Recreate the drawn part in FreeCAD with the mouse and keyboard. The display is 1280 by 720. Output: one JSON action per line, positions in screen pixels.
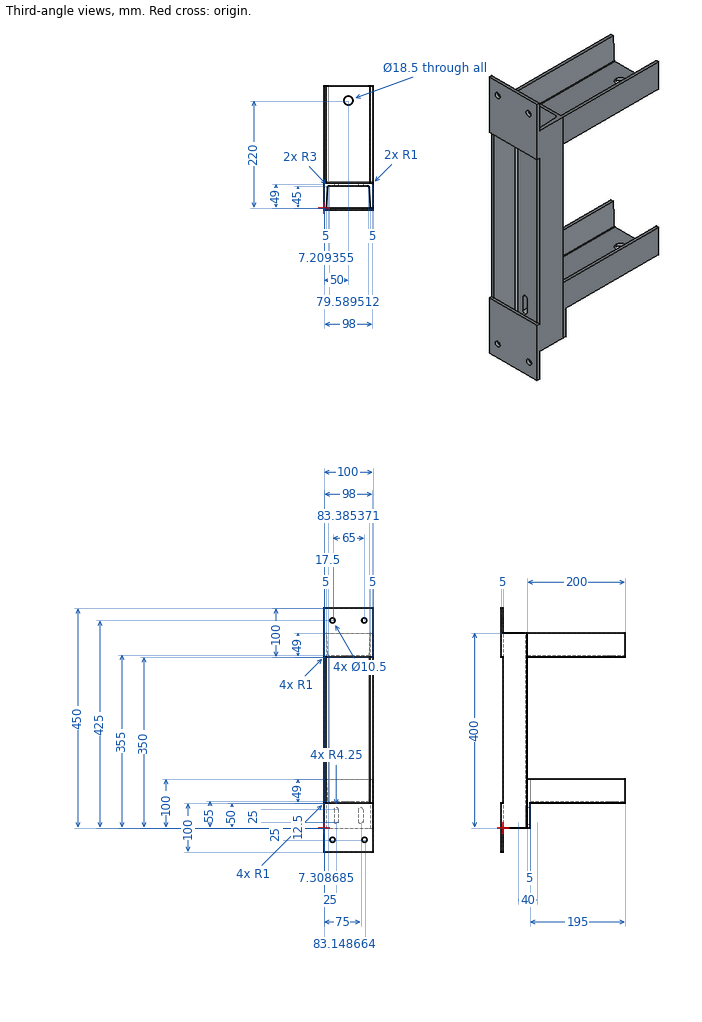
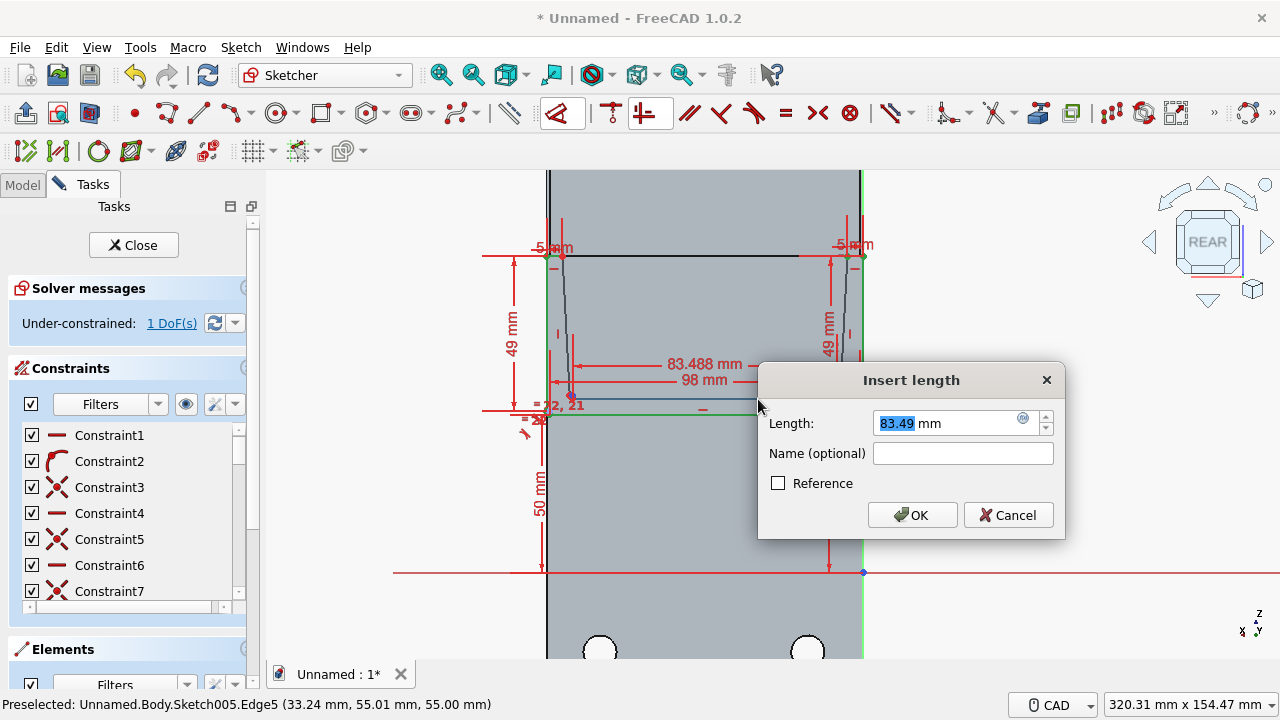
{"action": "type", "text": "83.385371"}
{"action": "key", "text": "Return"}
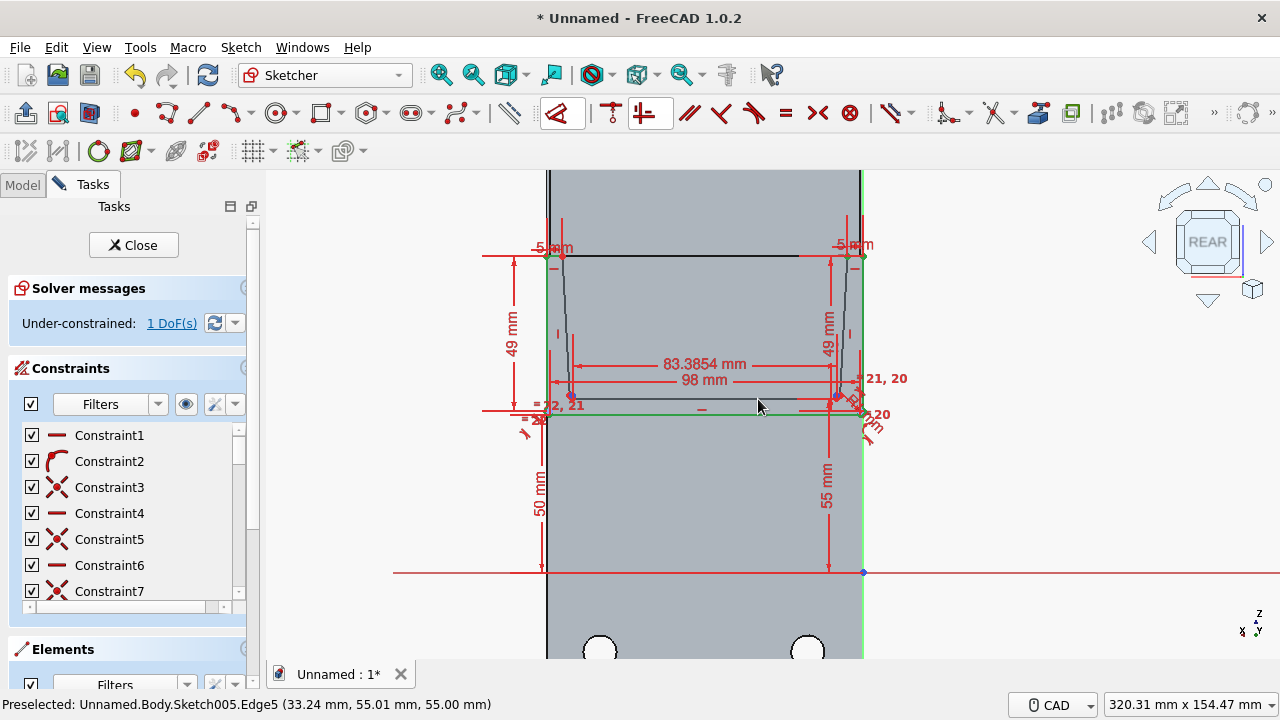
{"action": "scroll", "coordinate": [840, 396], "scroll_direction": "up", "scroll_amount": 7}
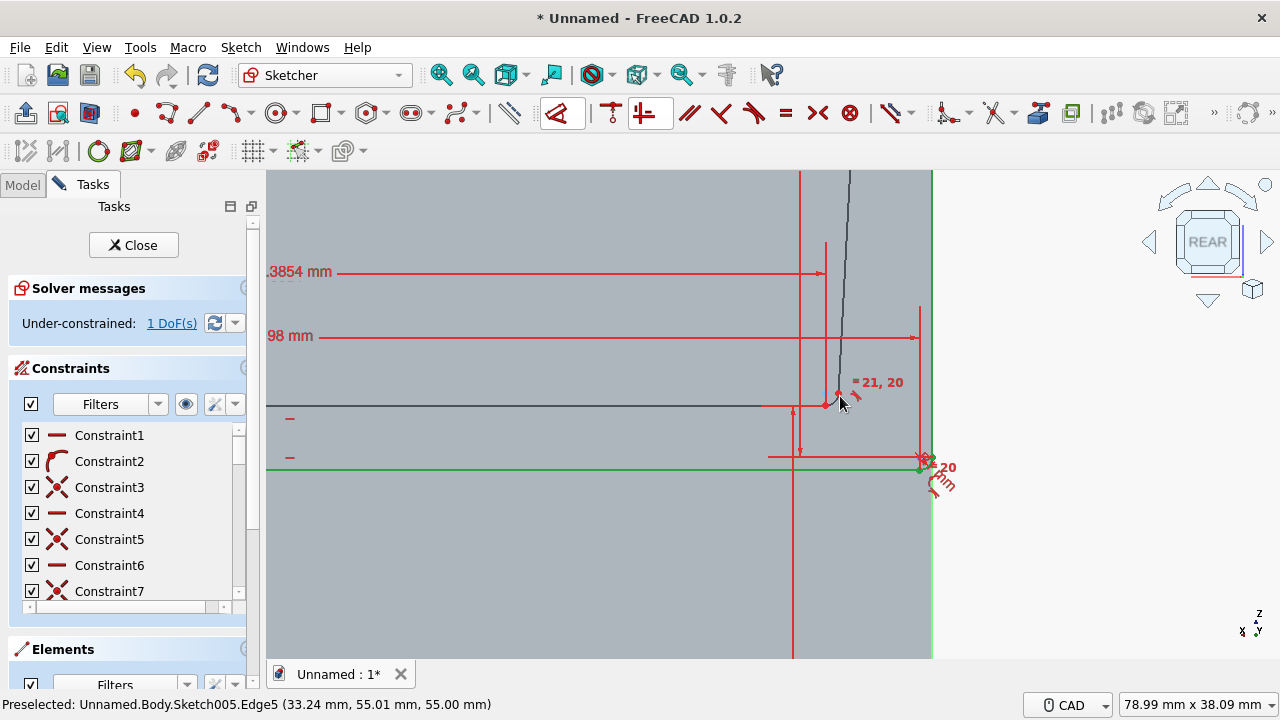
{"action": "left_click", "coordinate": [838, 394]}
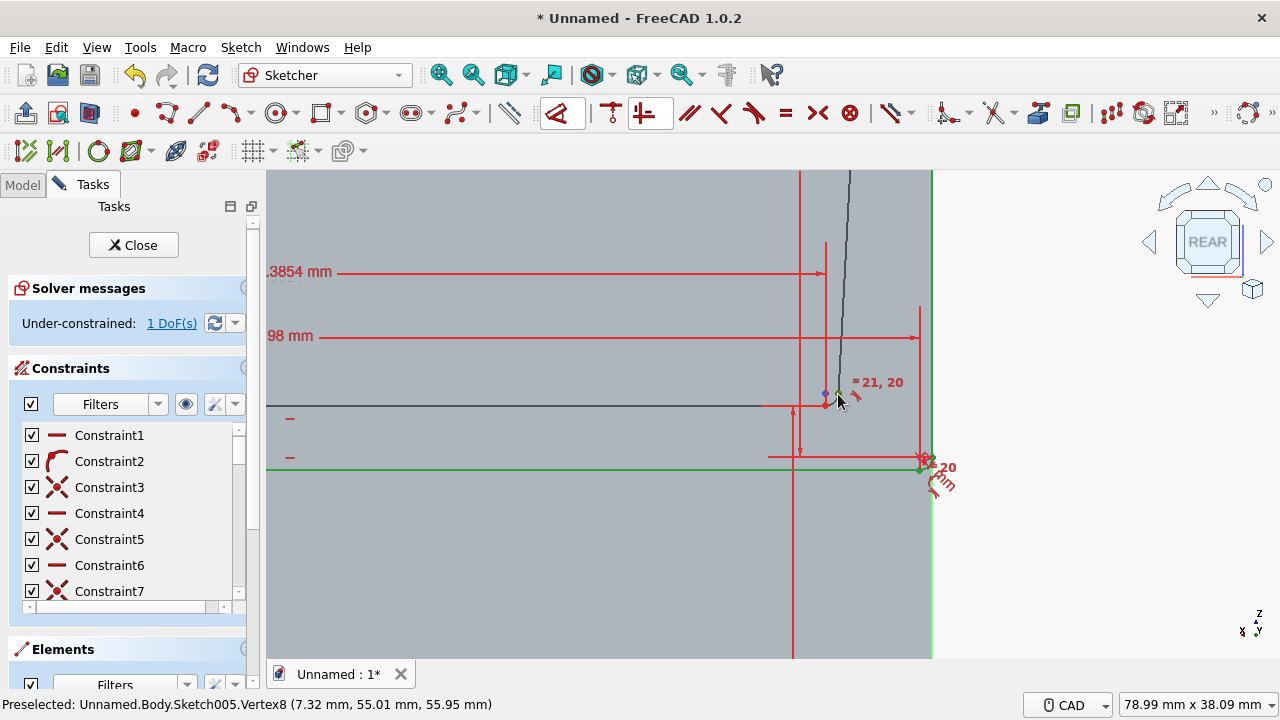
{"action": "key", "text": "l"}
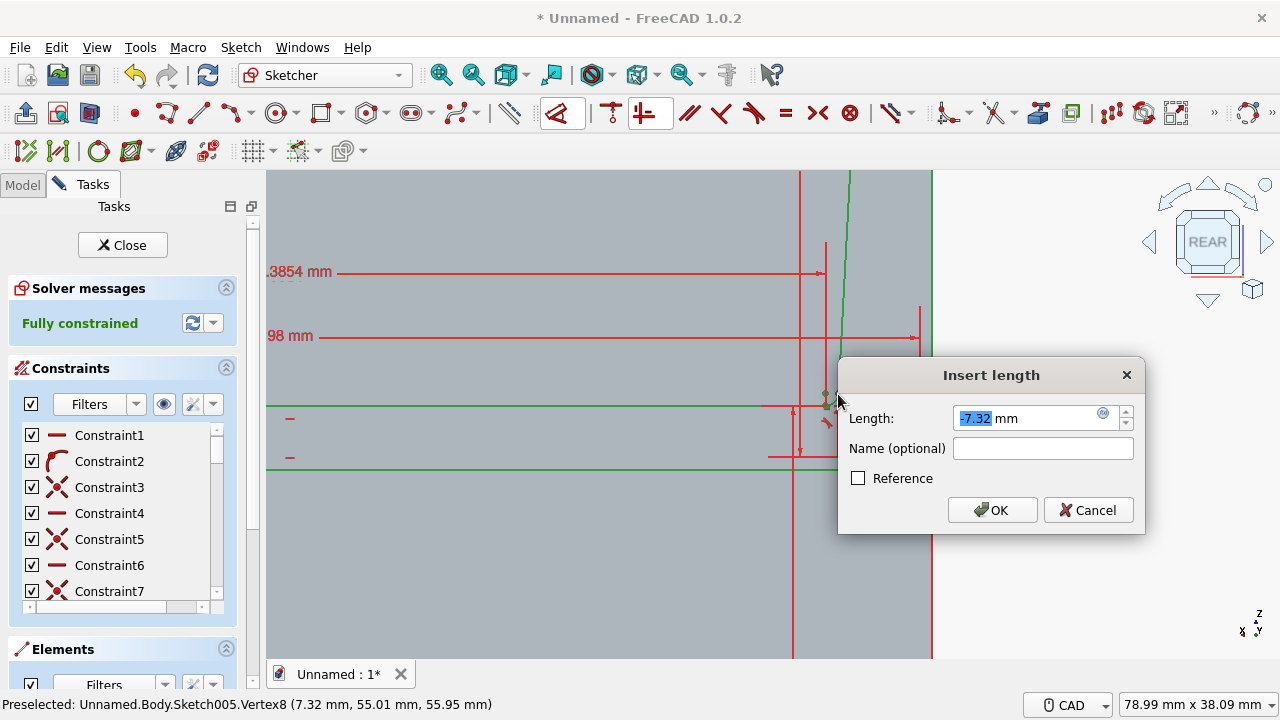
{"action": "type", "text": "-7.308685"}
{"action": "key", "text": "Return"}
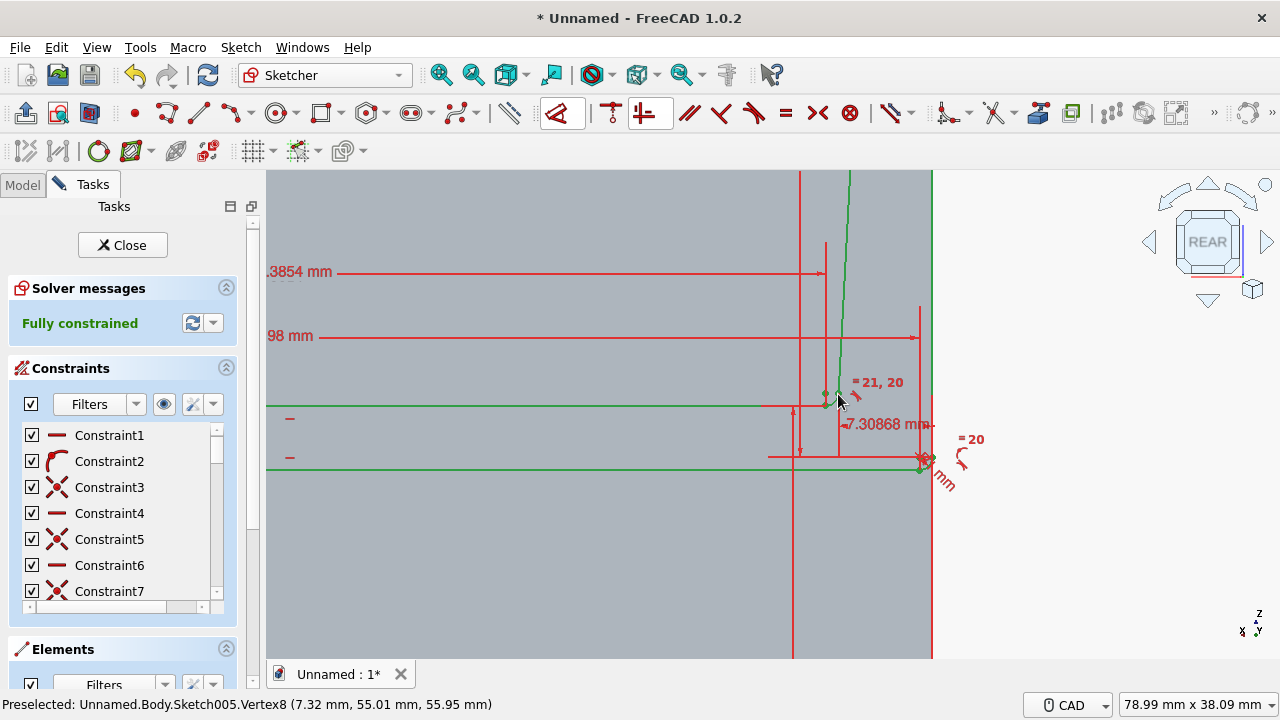
{"action": "left_click", "coordinate": [123, 245]}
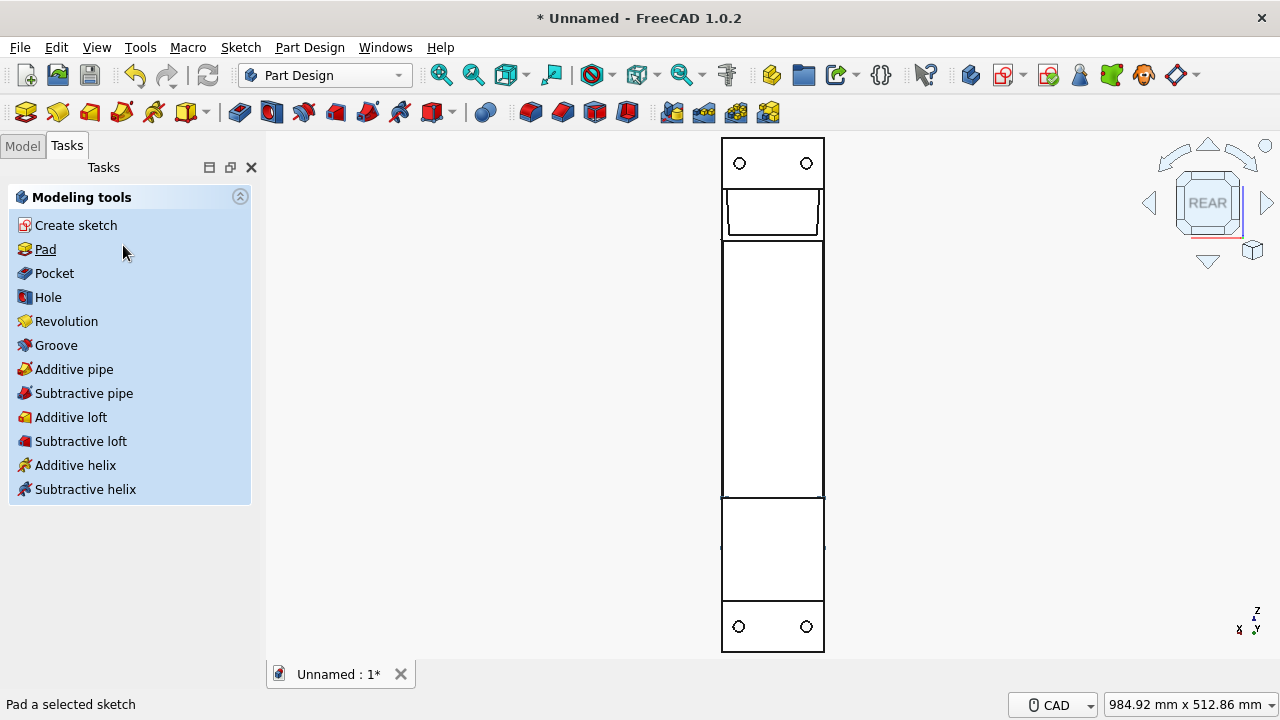
{"action": "left_click", "coordinate": [26, 112]}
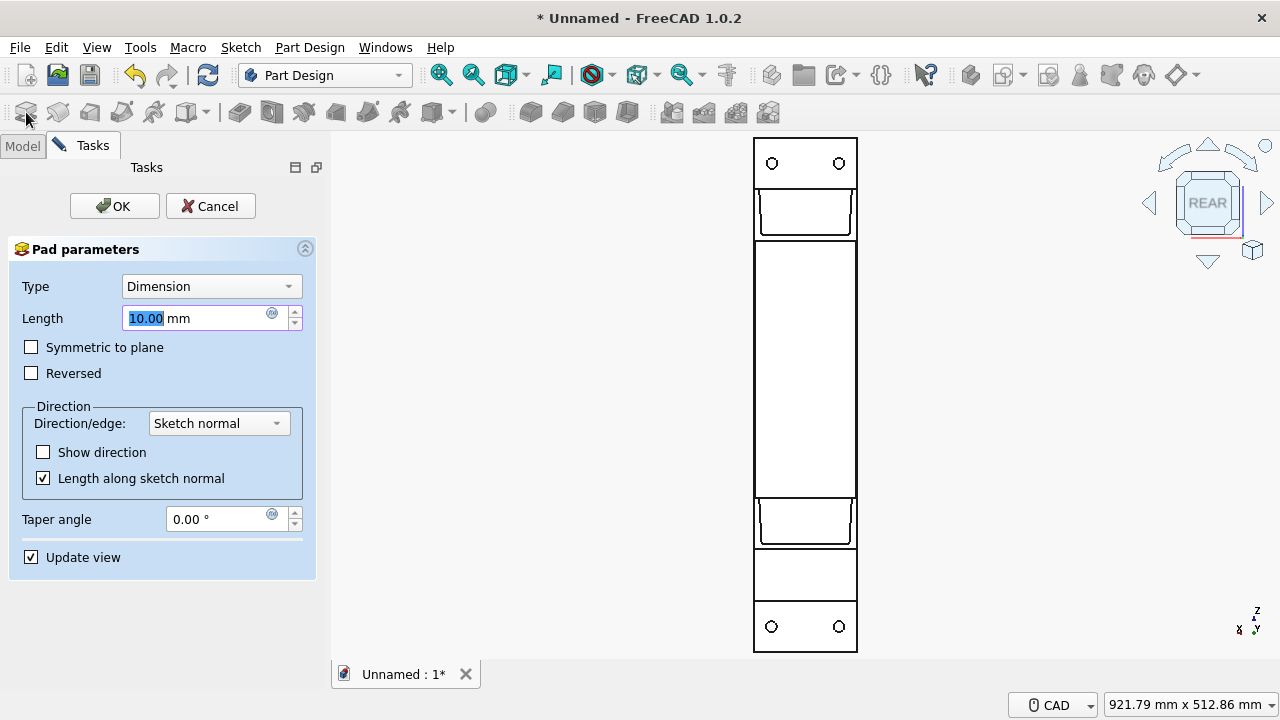
{"action": "type", "text": "195"}
{"action": "key", "text": "Tab"}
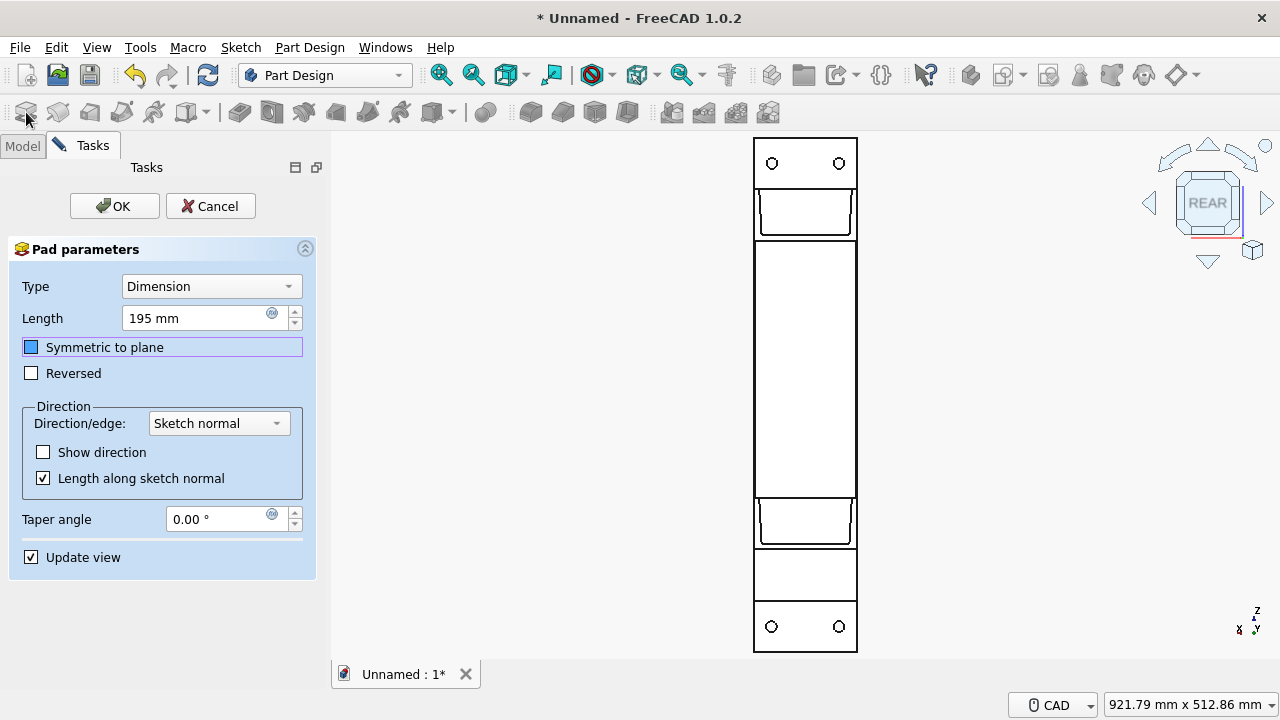
{"action": "left_click", "coordinate": [115, 206]}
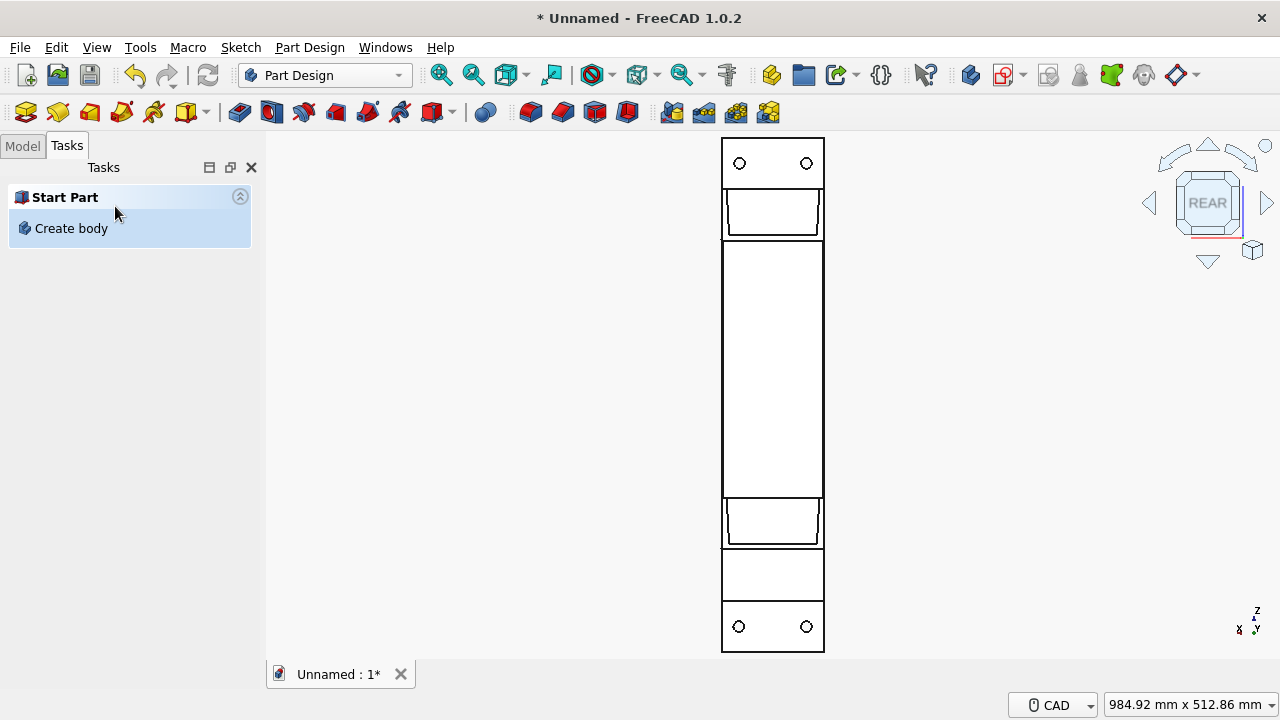
{"action": "left_click", "coordinate": [773, 295]}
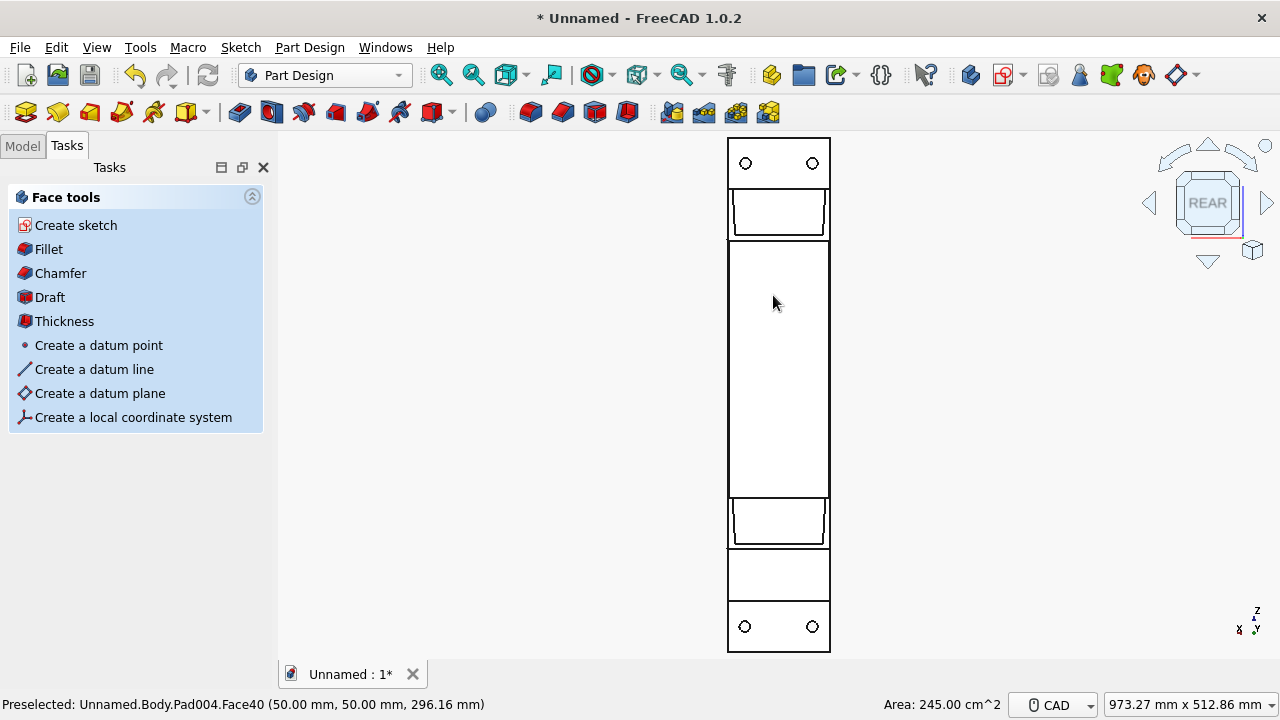
{"action": "left_click", "coordinate": [1004, 76]}